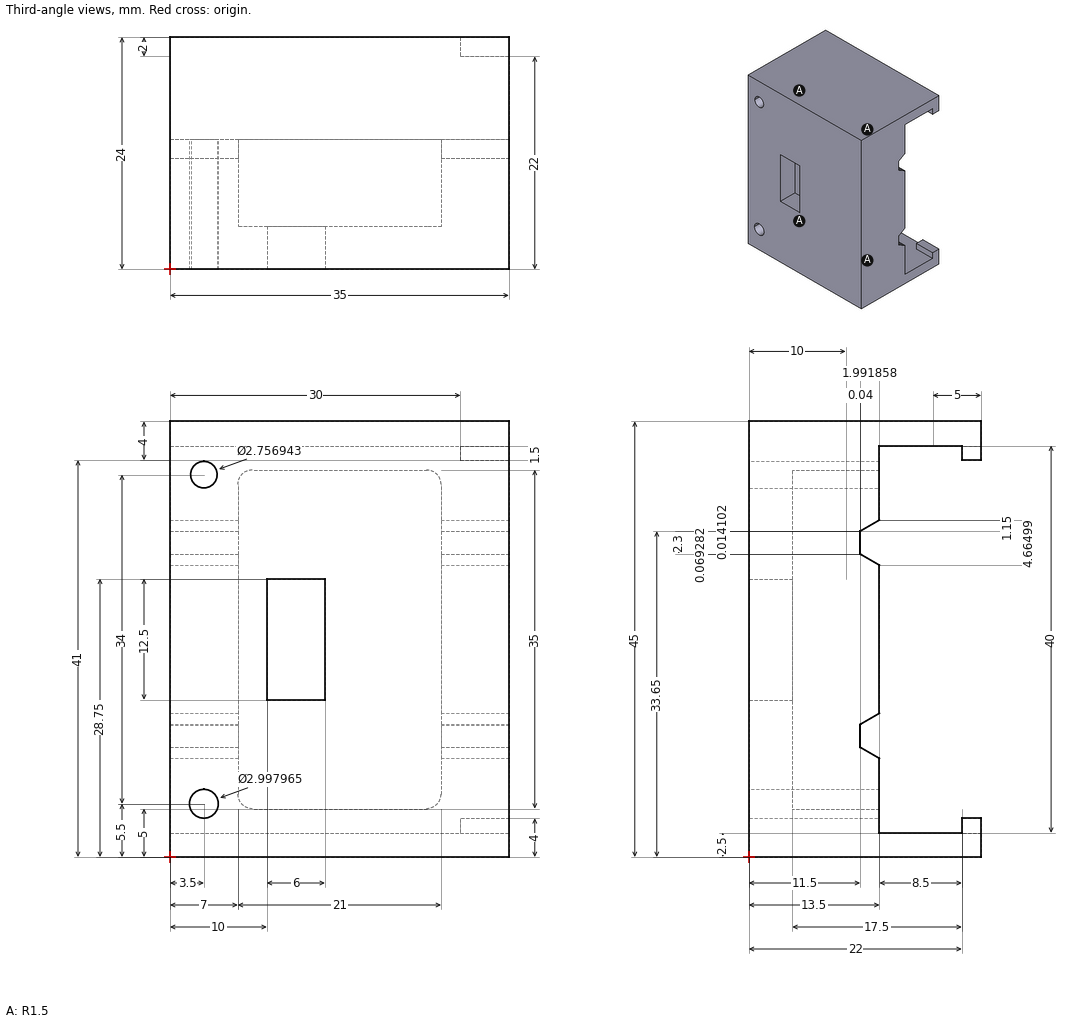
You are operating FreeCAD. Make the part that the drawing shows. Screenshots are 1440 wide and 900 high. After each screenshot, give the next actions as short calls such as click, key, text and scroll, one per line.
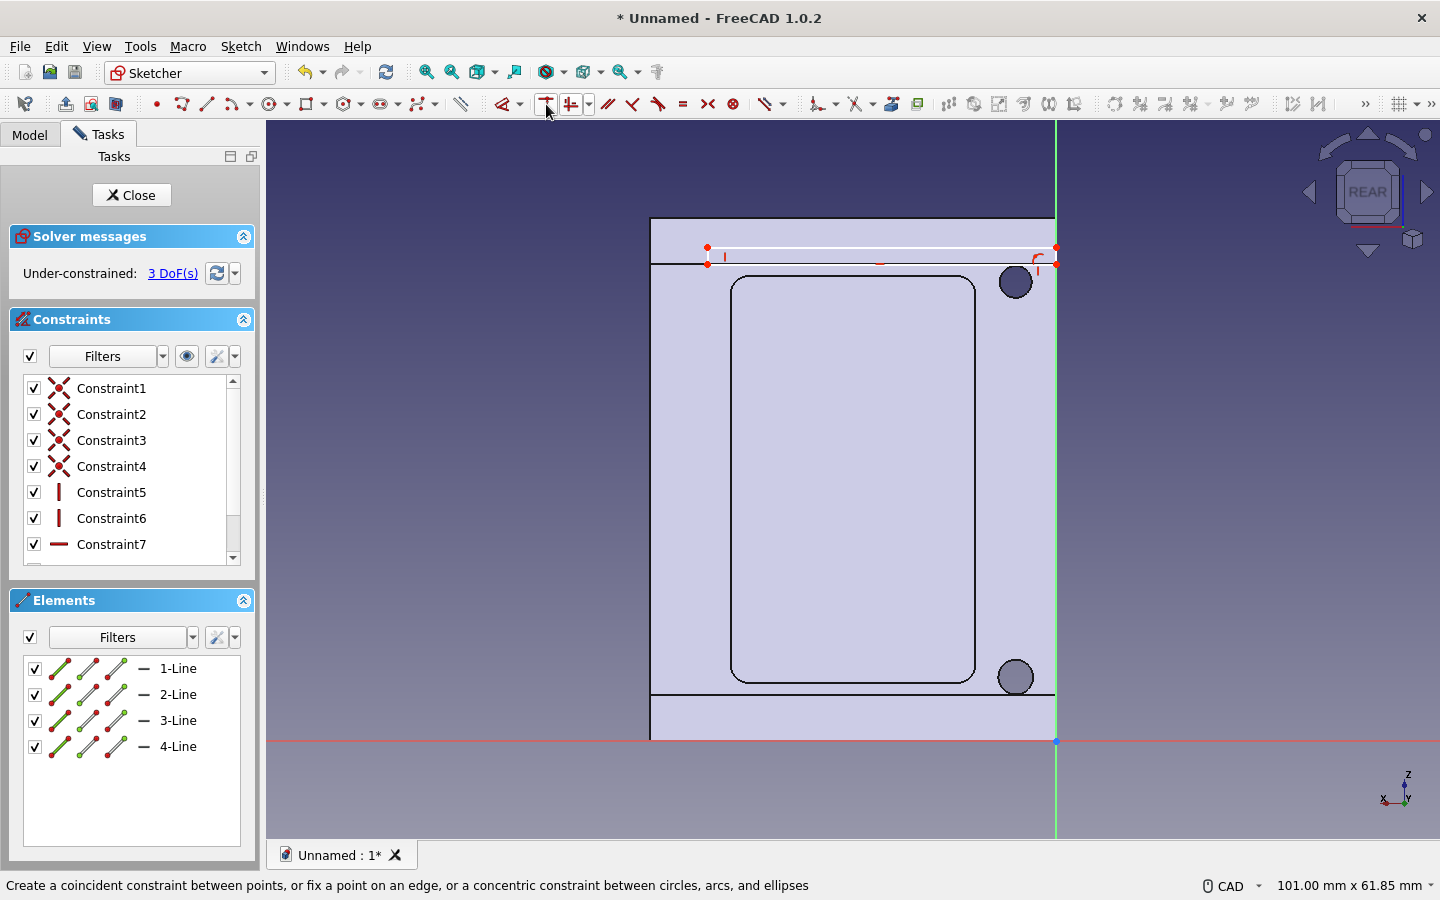
click(813, 265)
click(882, 231)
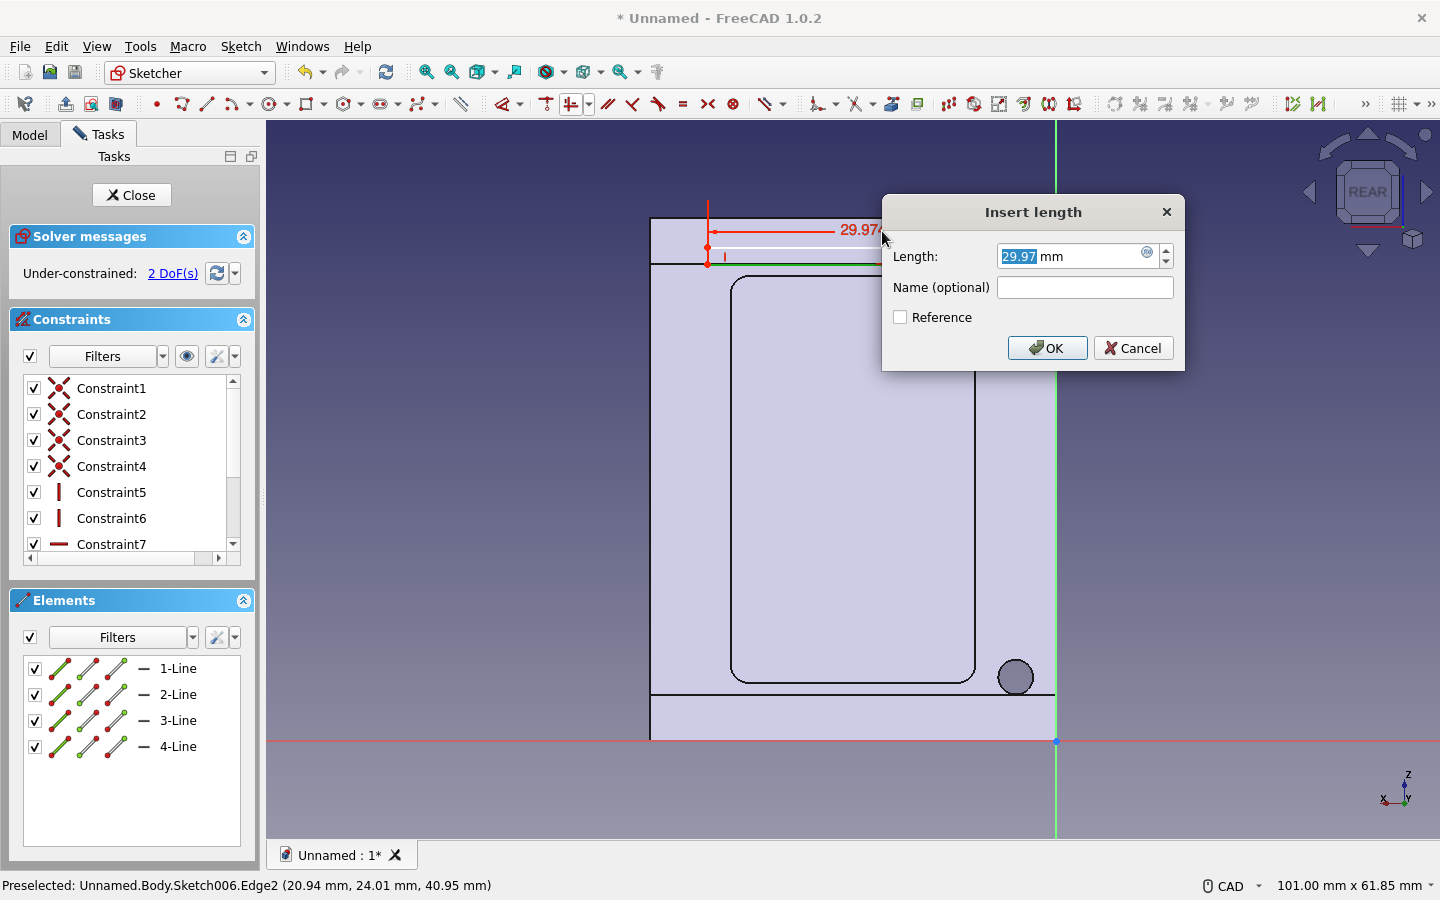
text(30)
key(Return)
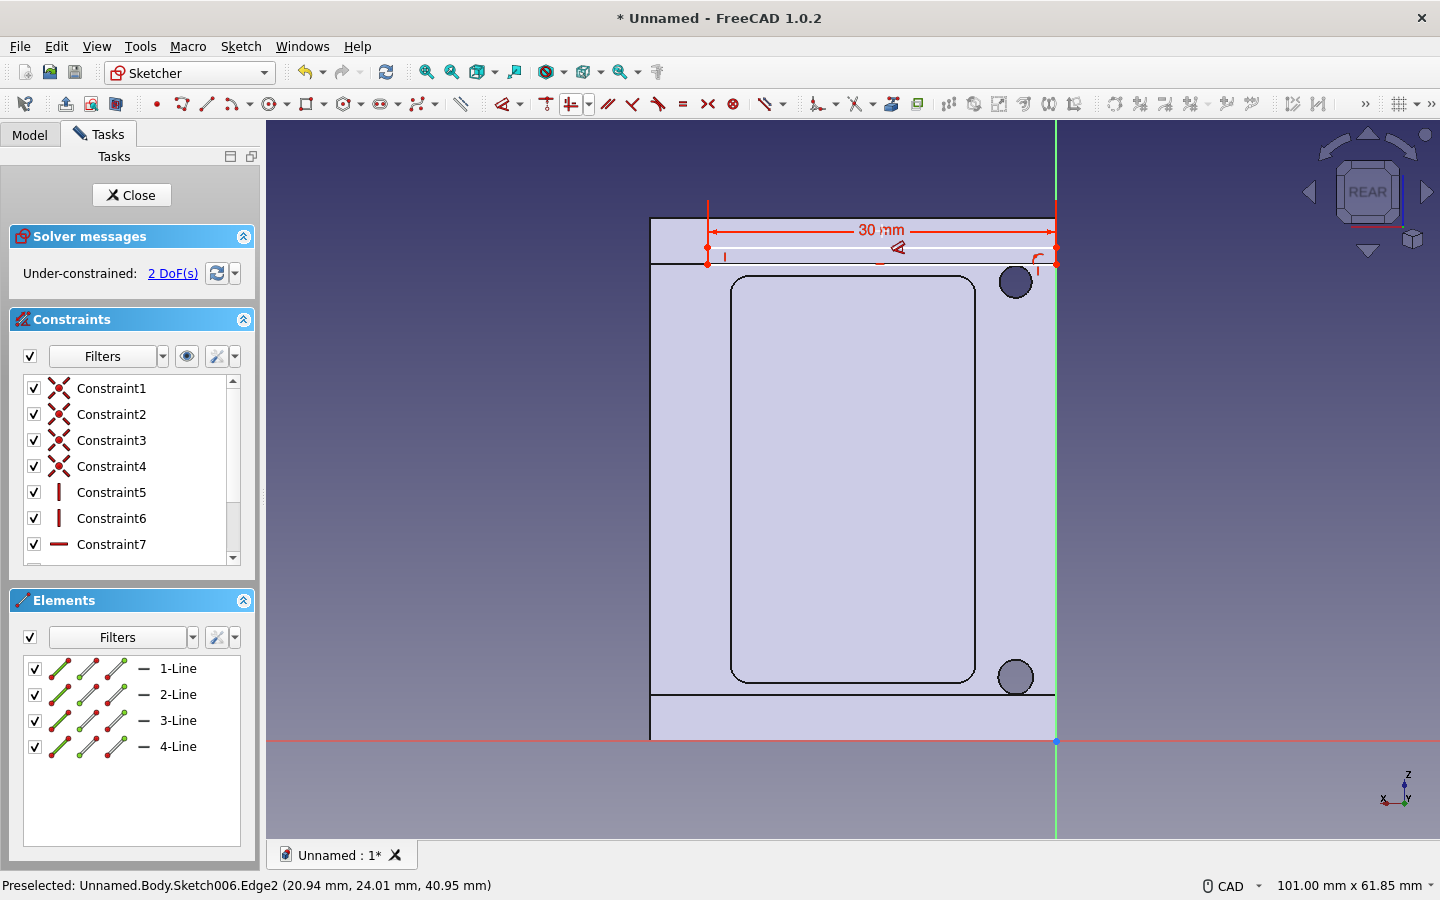
scroll(708, 256, up, 5)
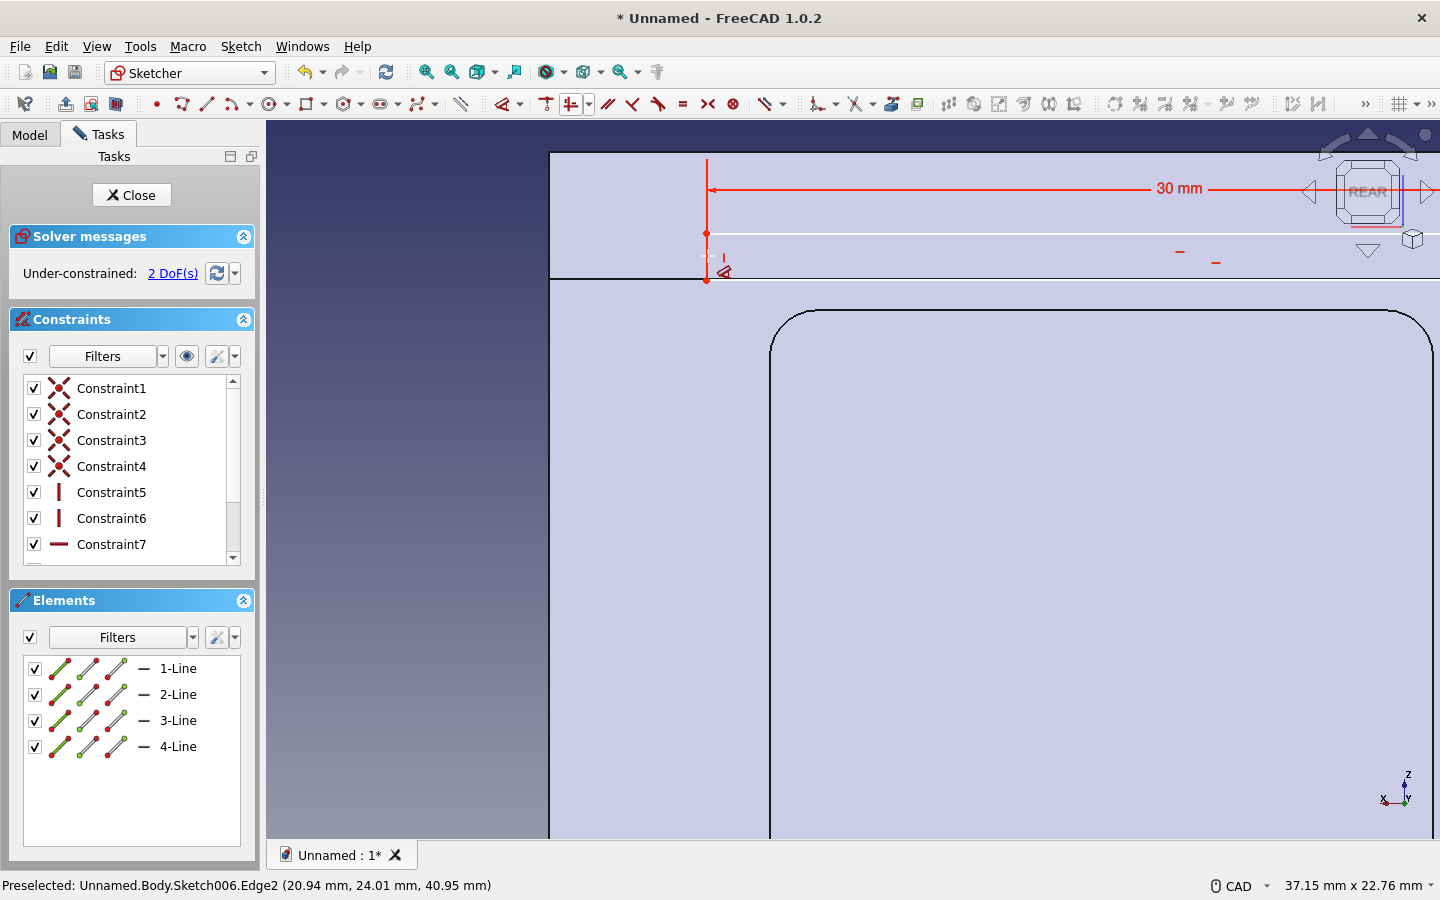
click(707, 257)
click(673, 257)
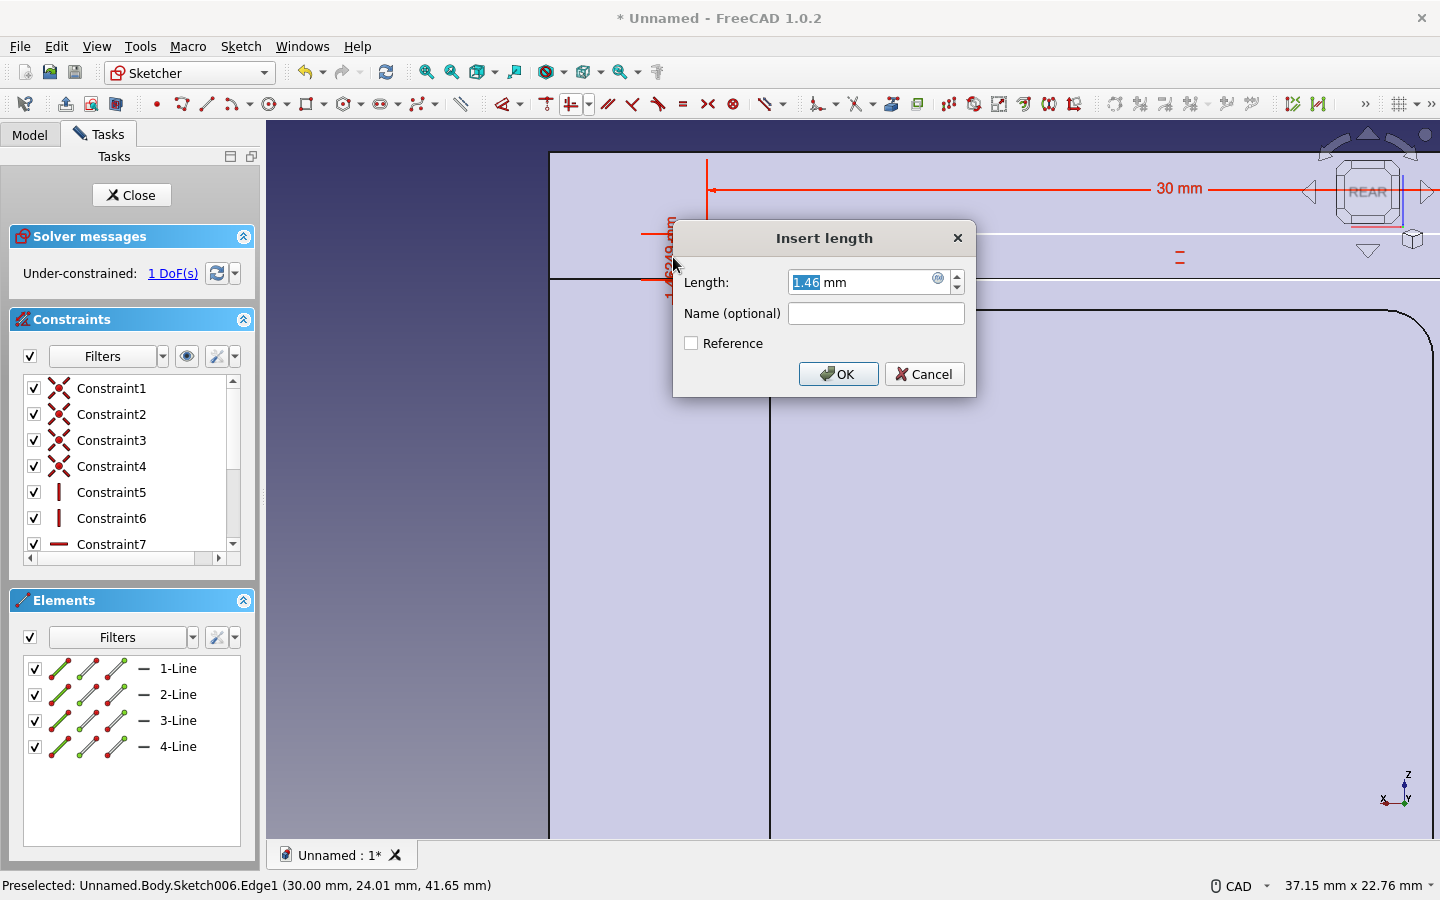
text(1.5)
key(Return)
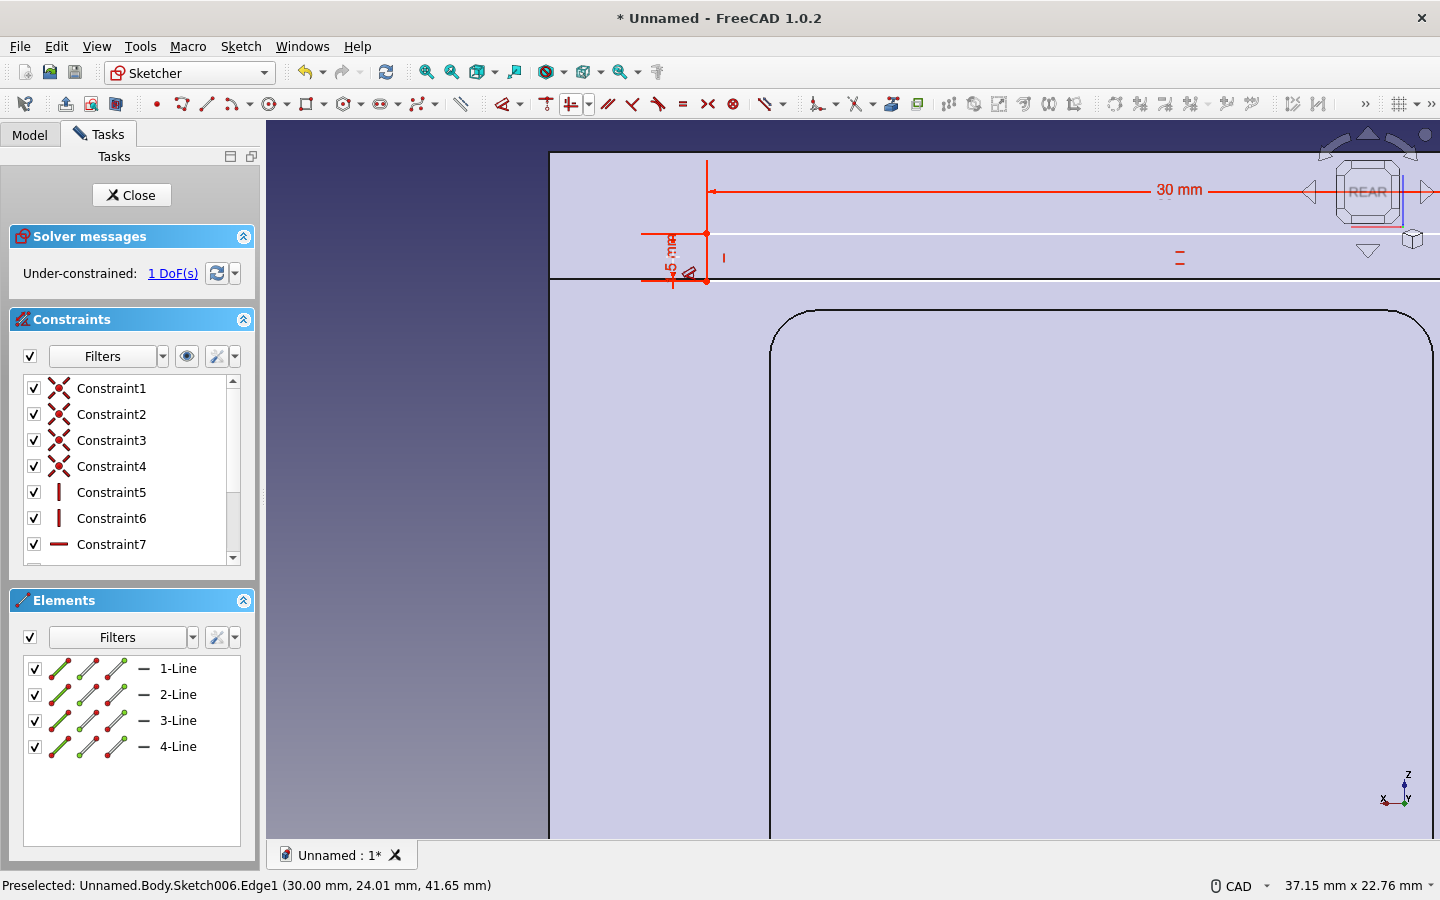
click(707, 281)
click(673, 546)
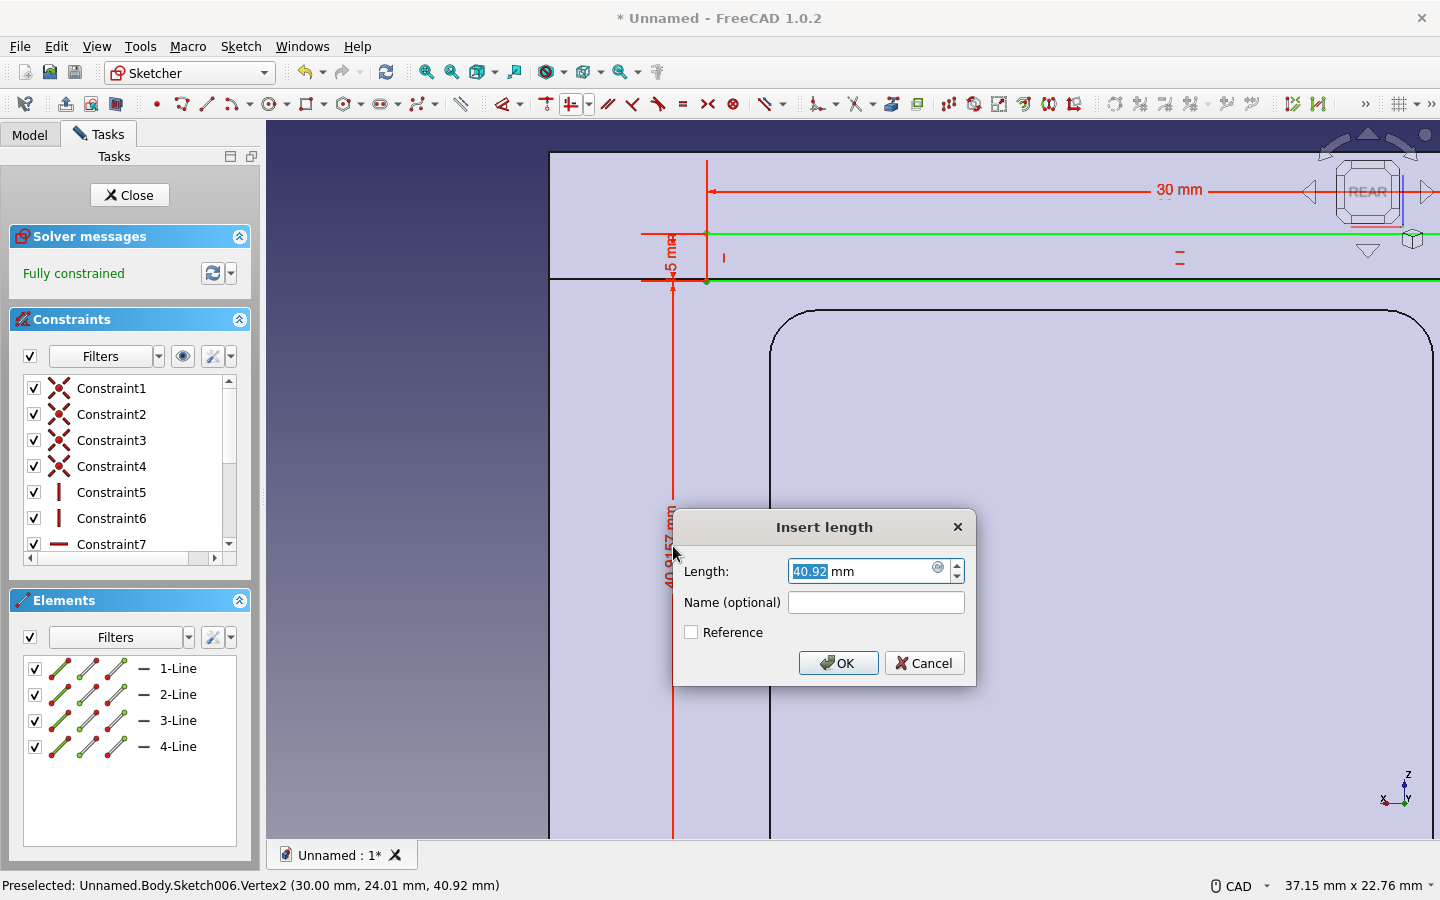
text(41)
key(Return)
key(Escape)